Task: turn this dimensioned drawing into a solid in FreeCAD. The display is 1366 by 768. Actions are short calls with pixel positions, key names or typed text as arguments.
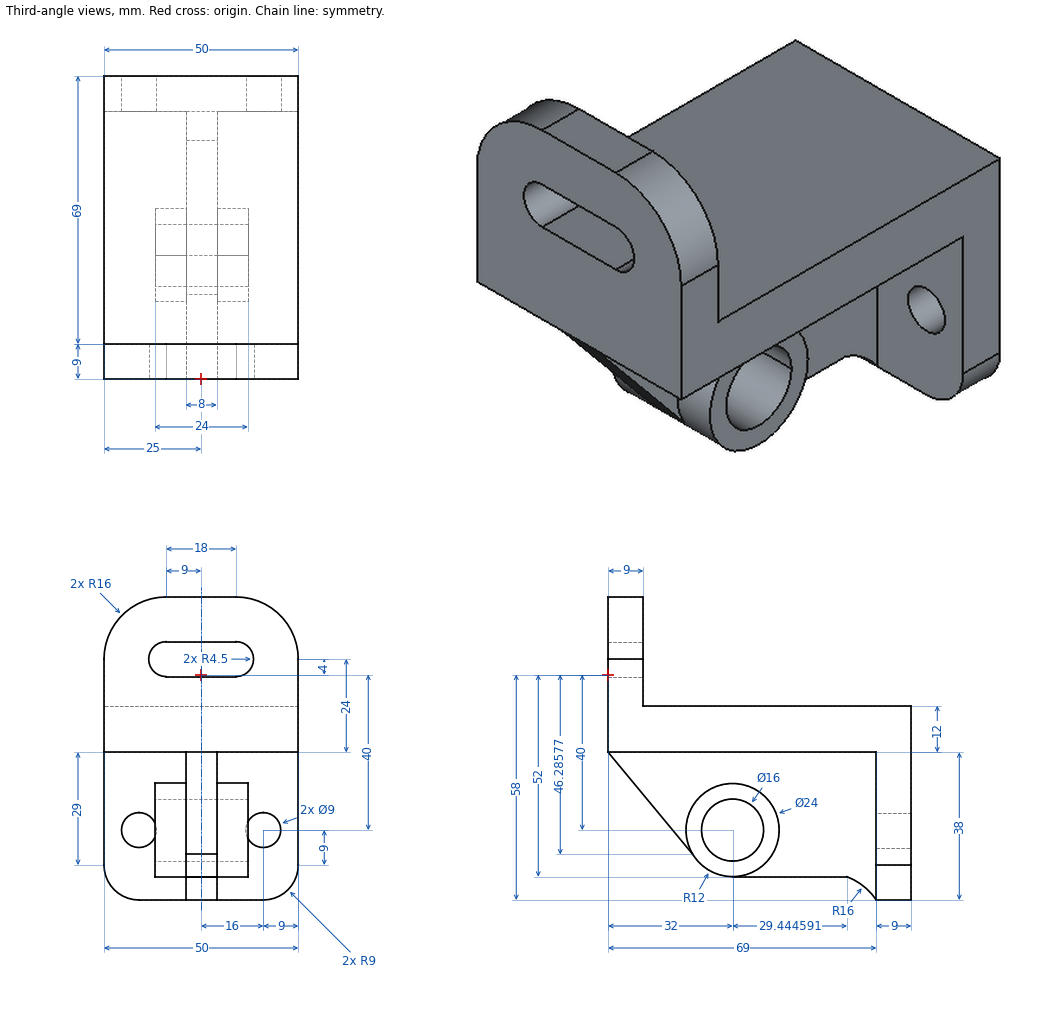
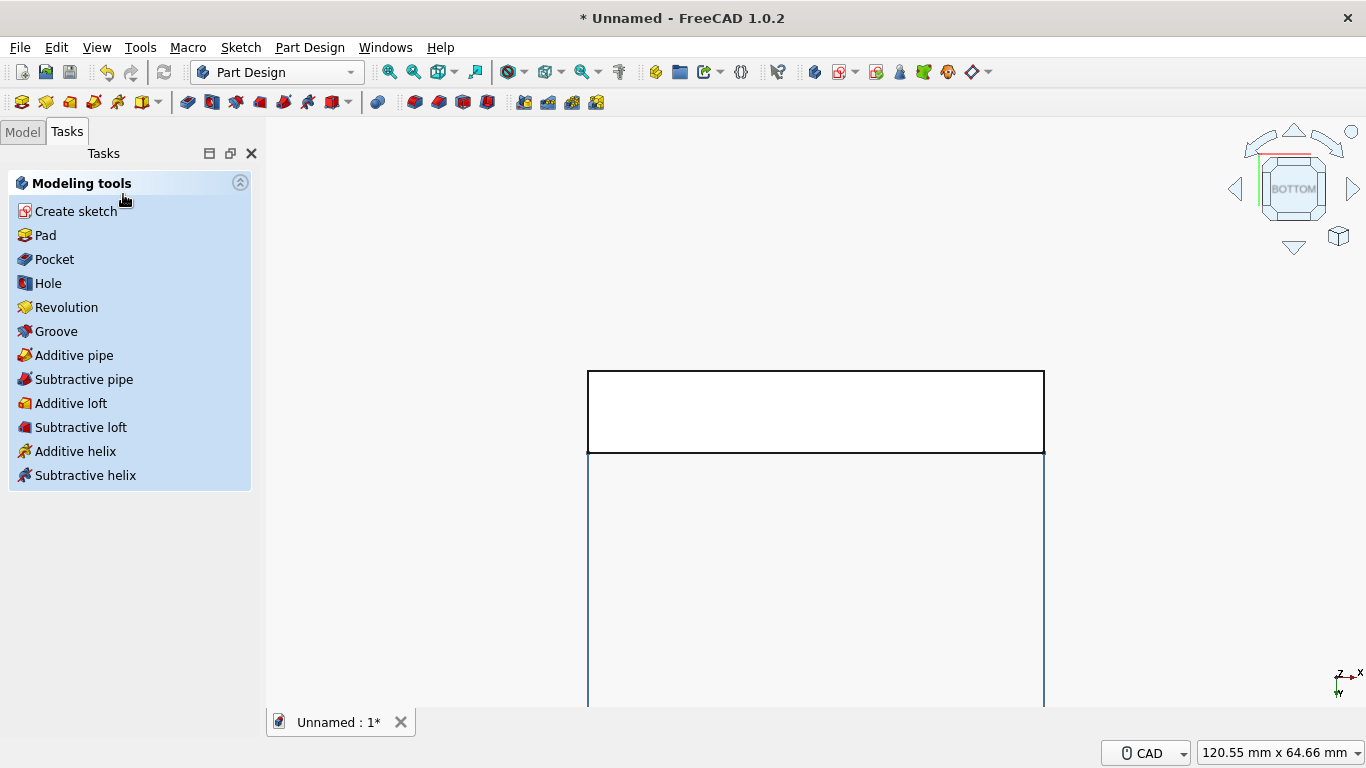
click(22, 102)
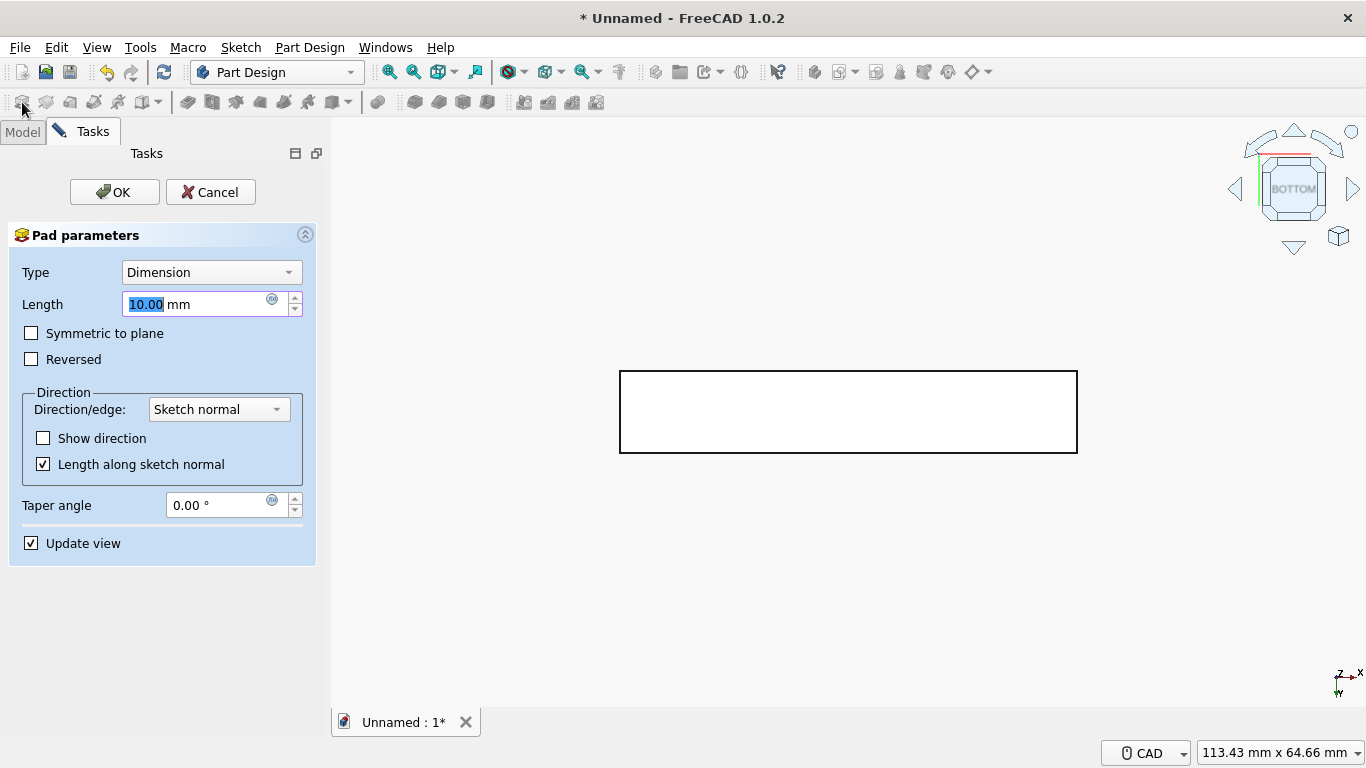
text(12)
key(Tab)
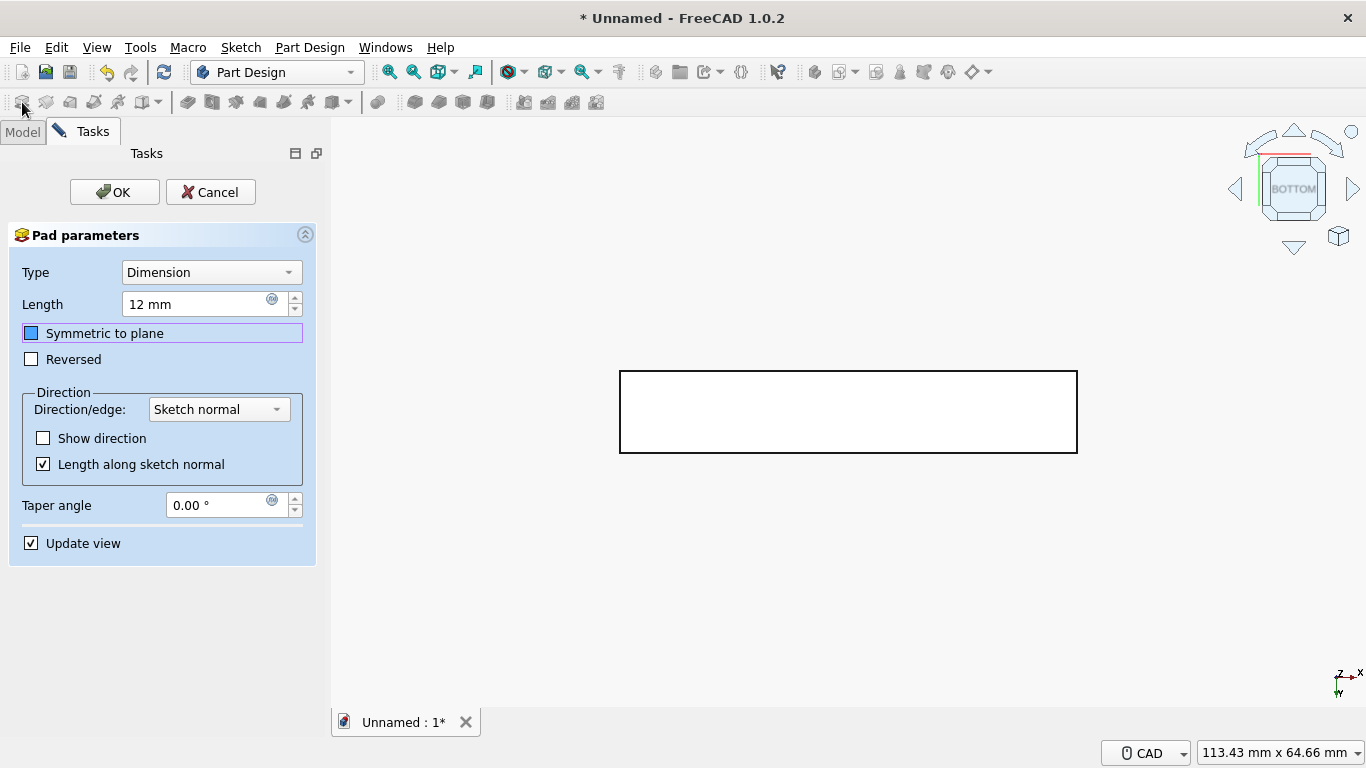
click(30, 359)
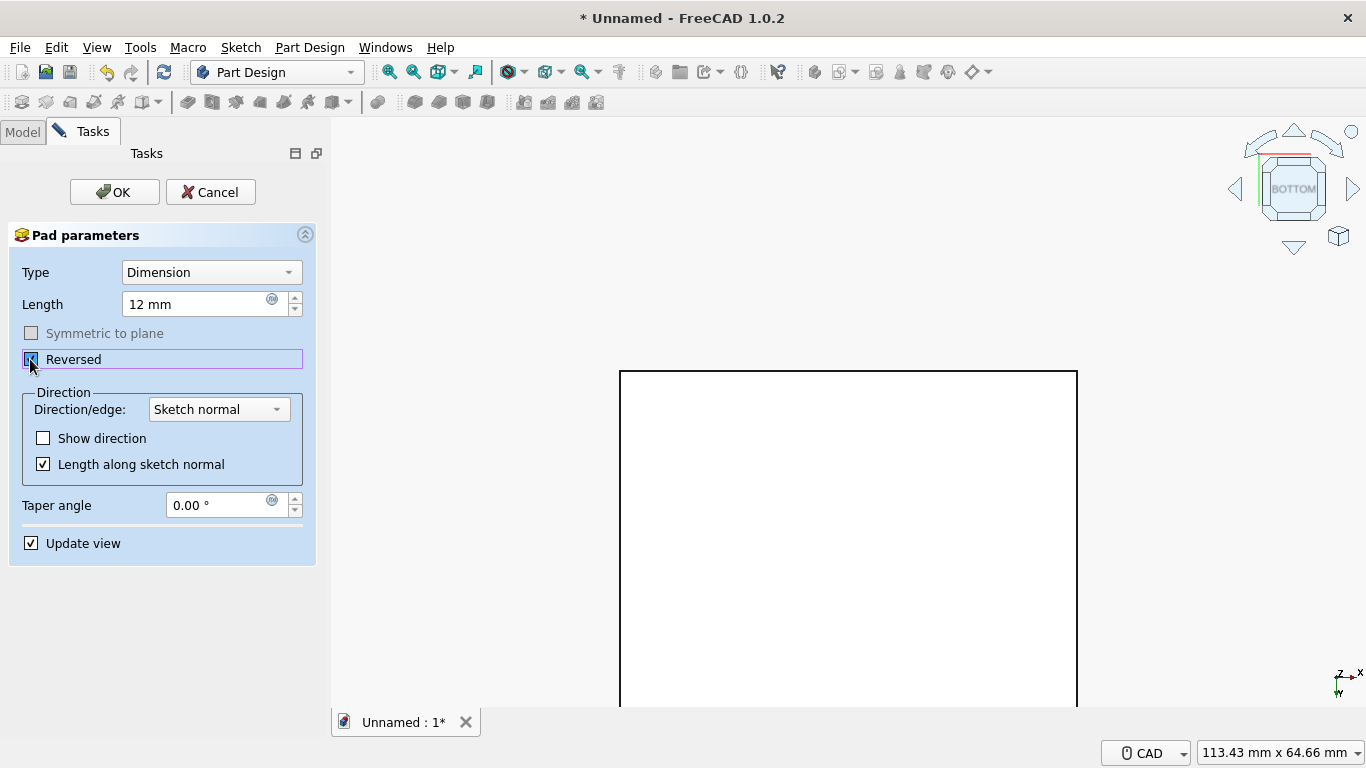
click(115, 192)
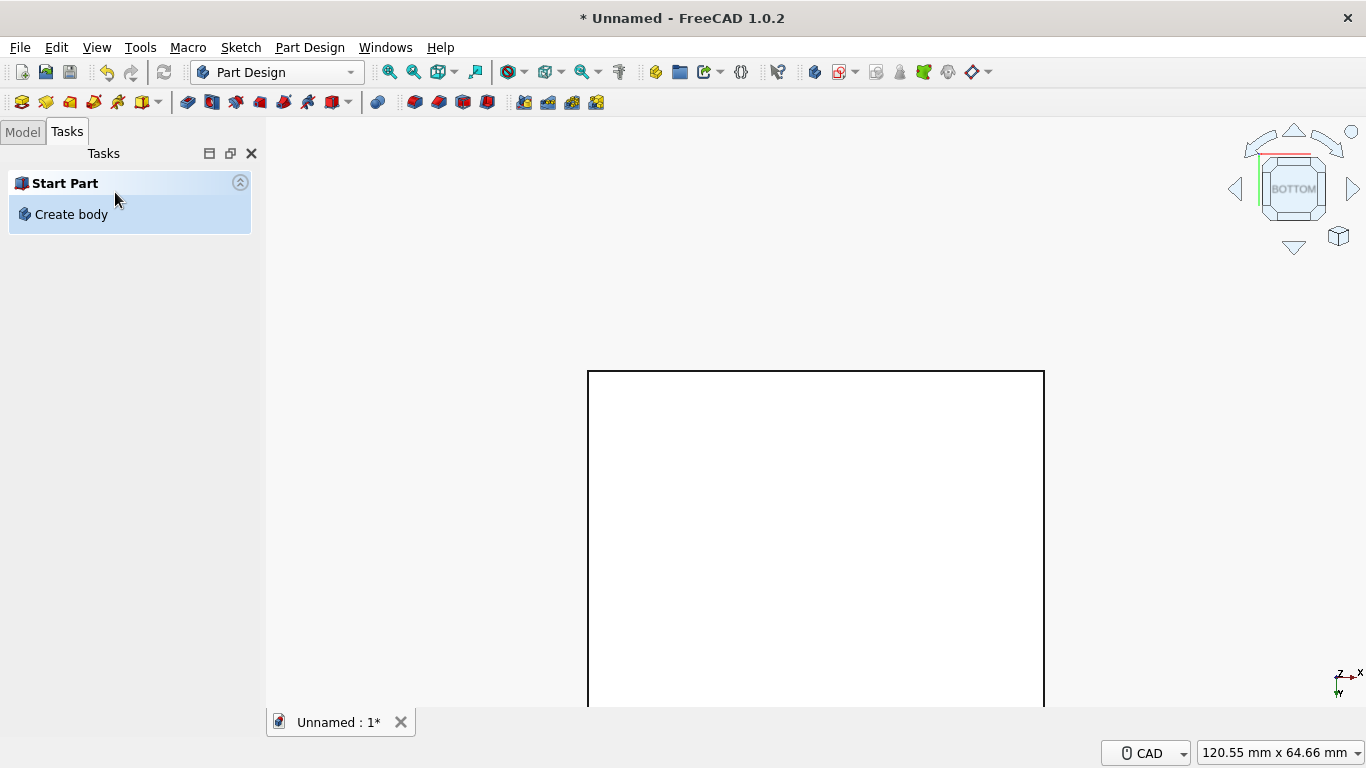
click(390, 72)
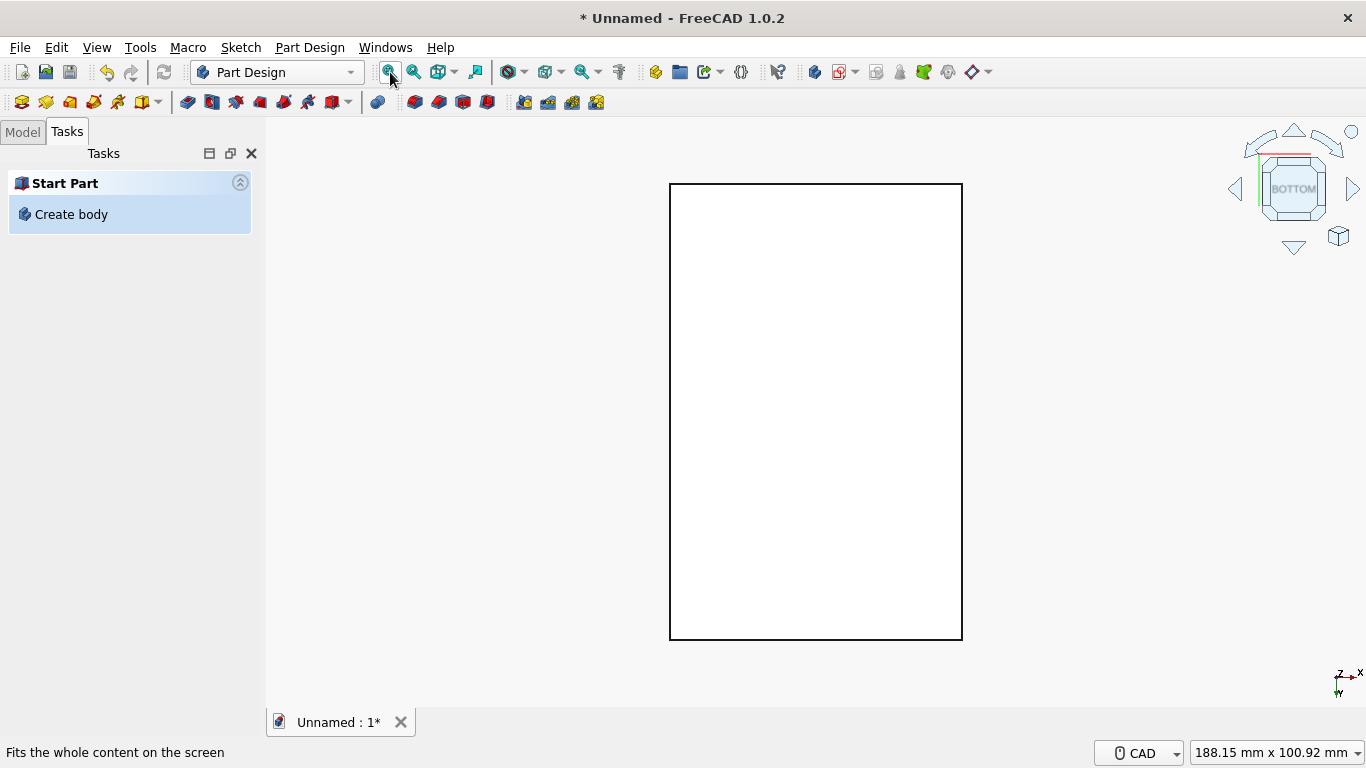
key(4)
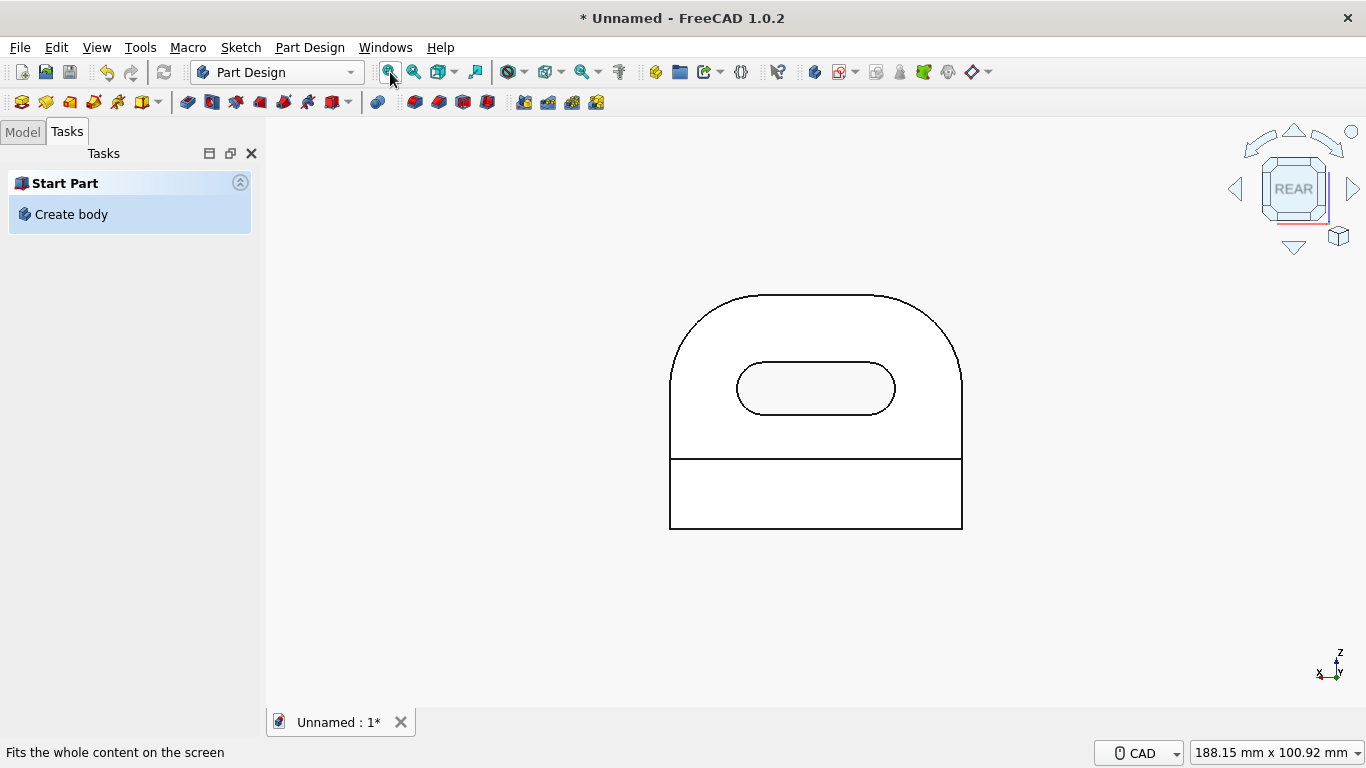
click(390, 72)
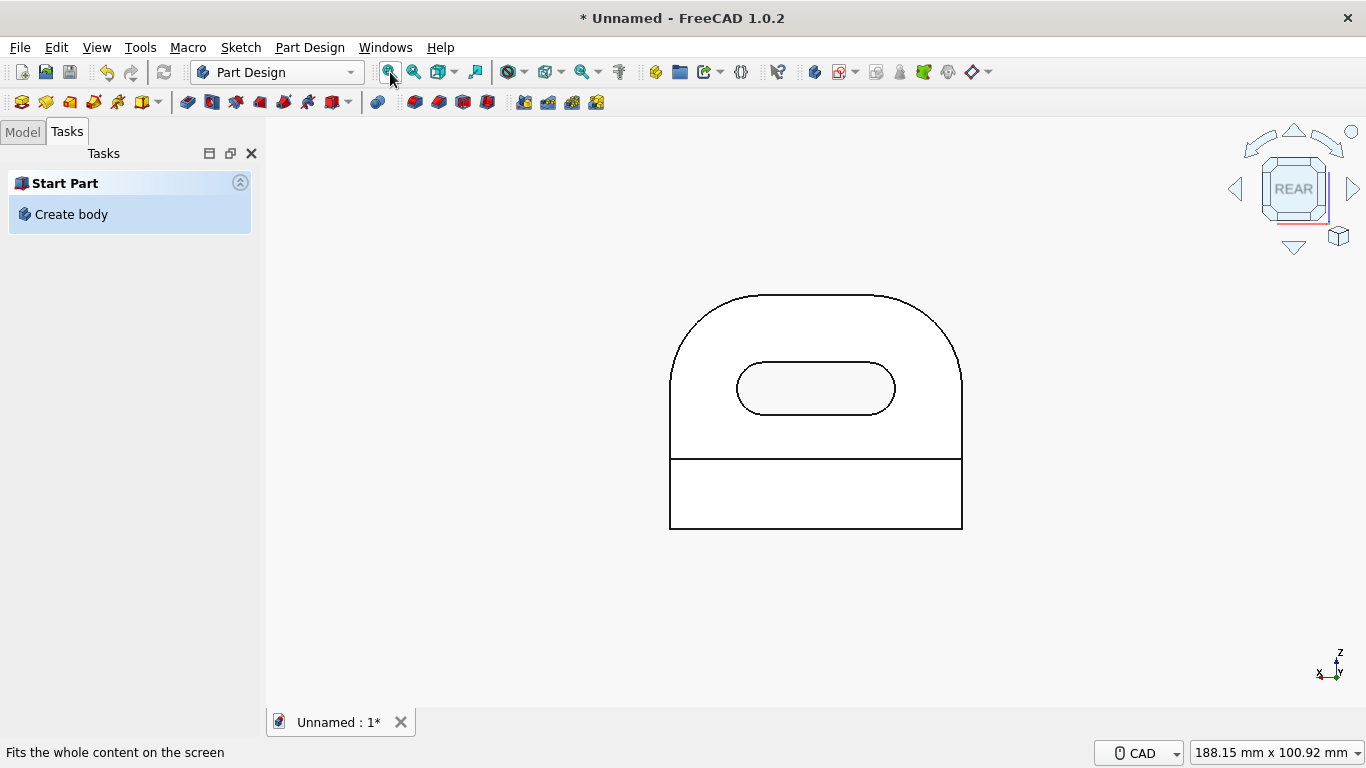
click(732, 493)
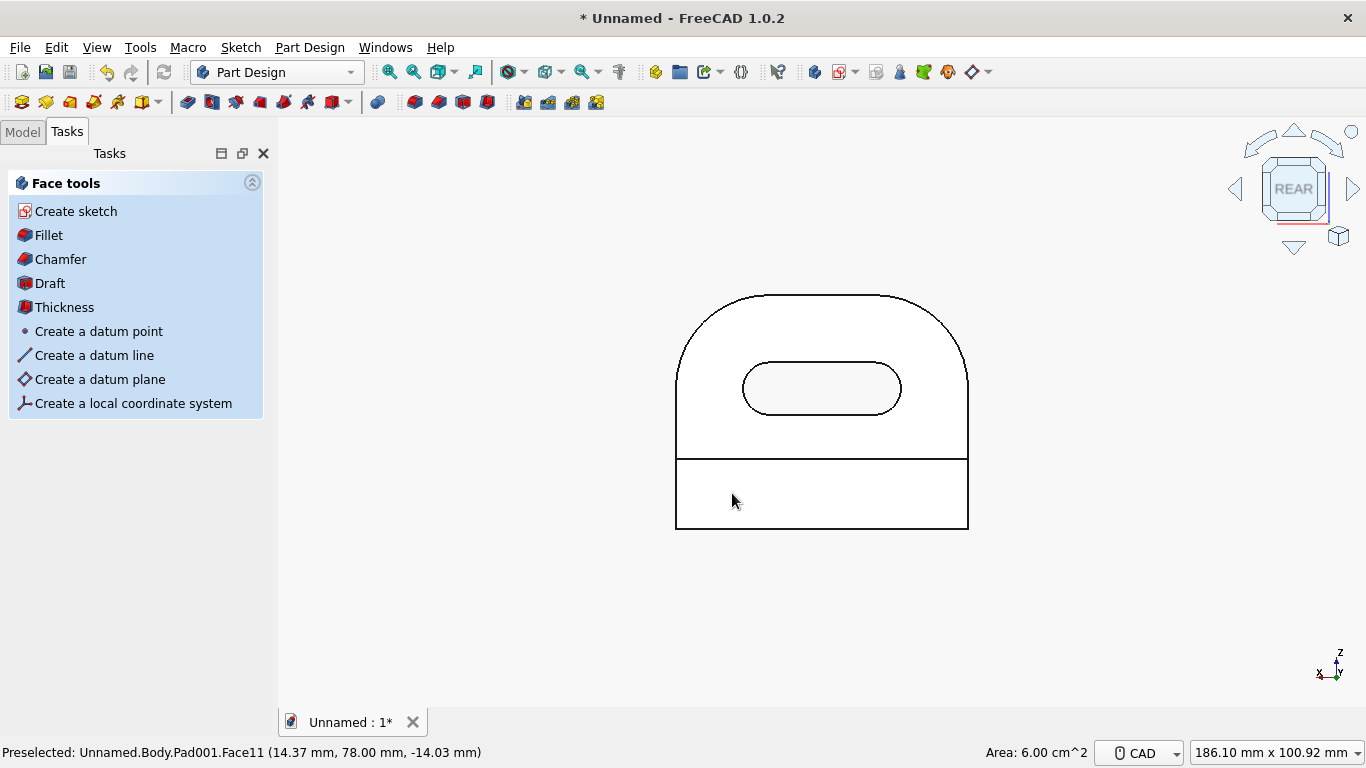
click(840, 72)